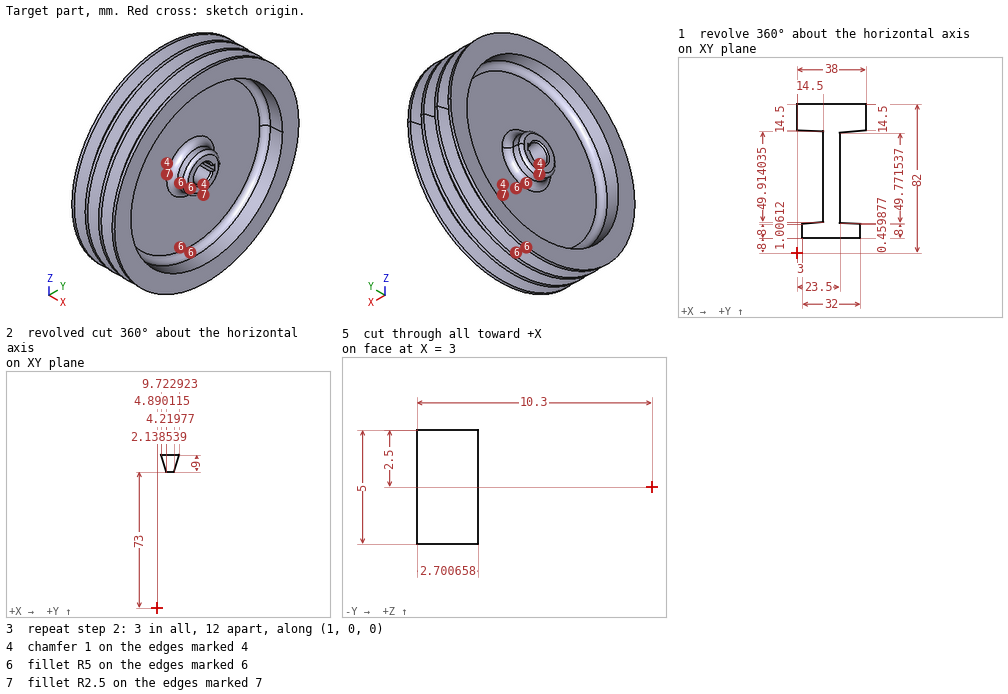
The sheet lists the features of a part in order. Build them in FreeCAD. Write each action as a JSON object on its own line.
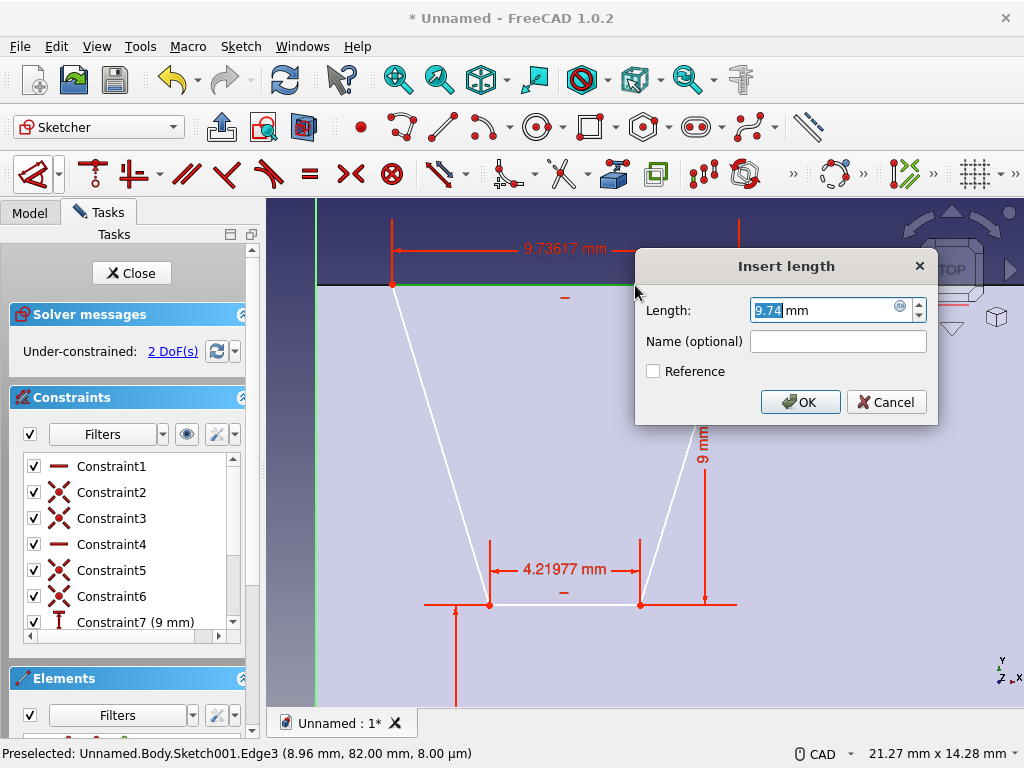
{"action": "type", "text": "9.722923"}
{"action": "key", "text": "Return"}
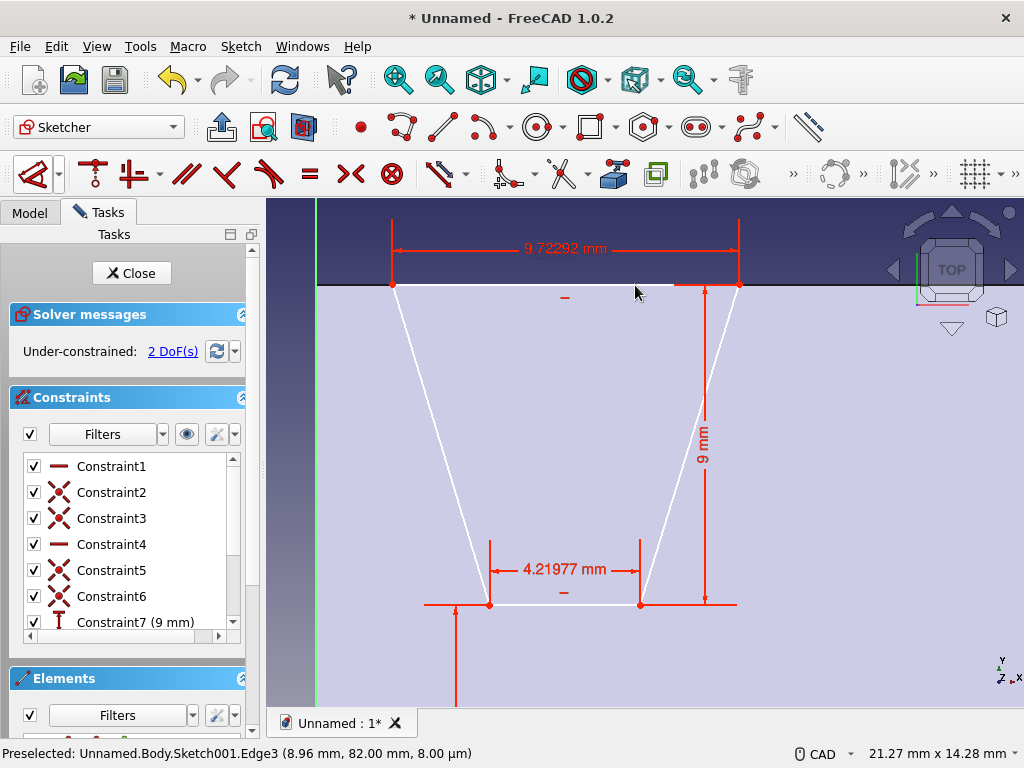
{"action": "left_click", "coordinate": [490, 605]}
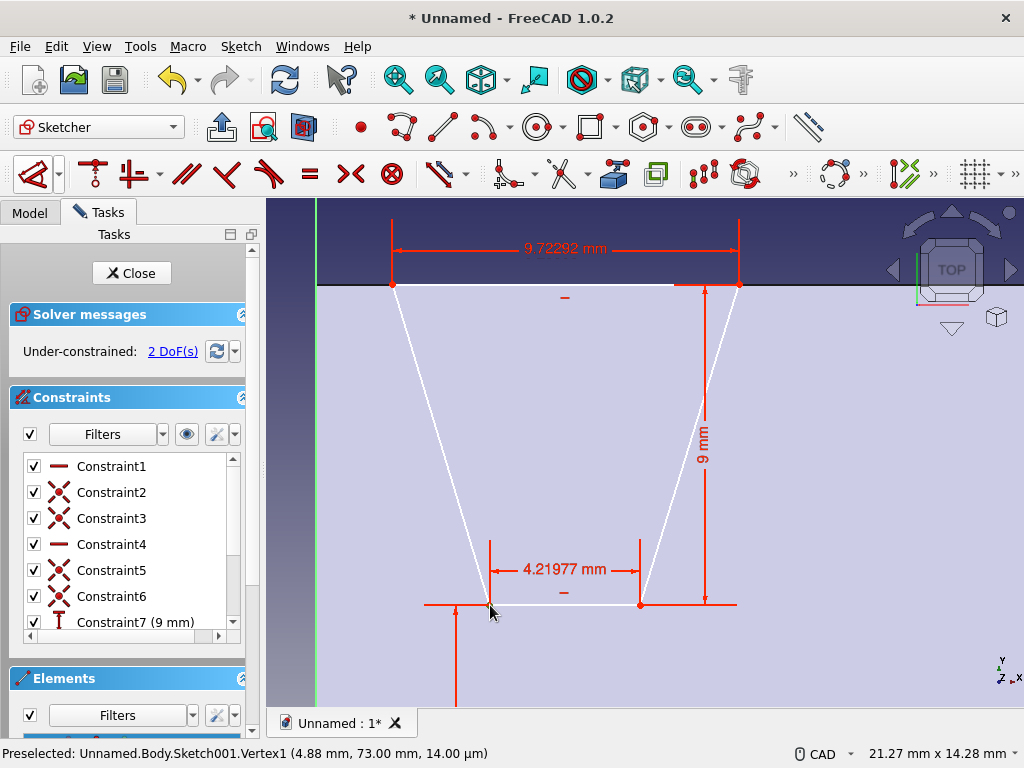
{"action": "key", "text": "l"}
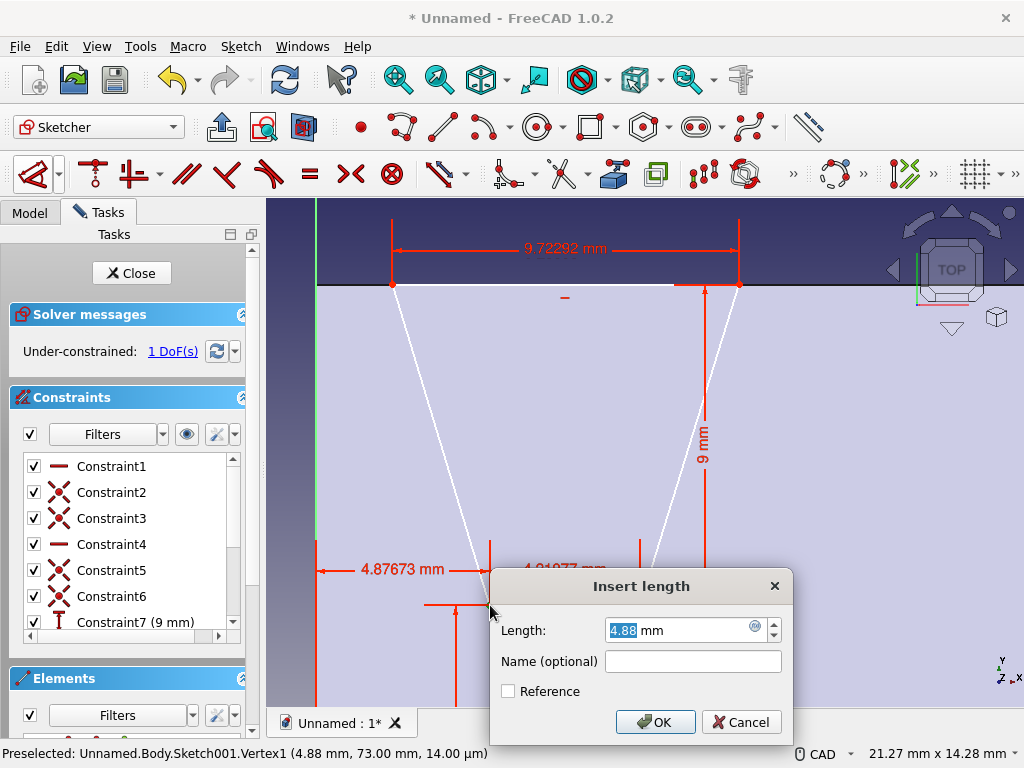
{"action": "type", "text": "4.890115"}
{"action": "key", "text": "Return"}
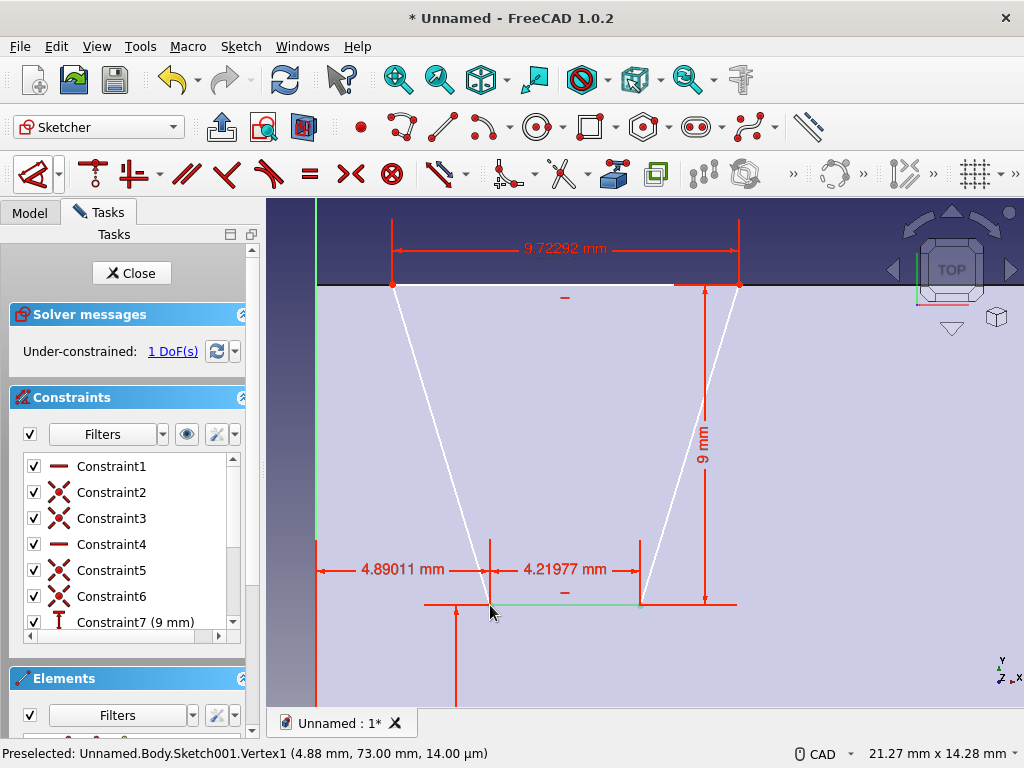
{"action": "left_click", "coordinate": [392, 285]}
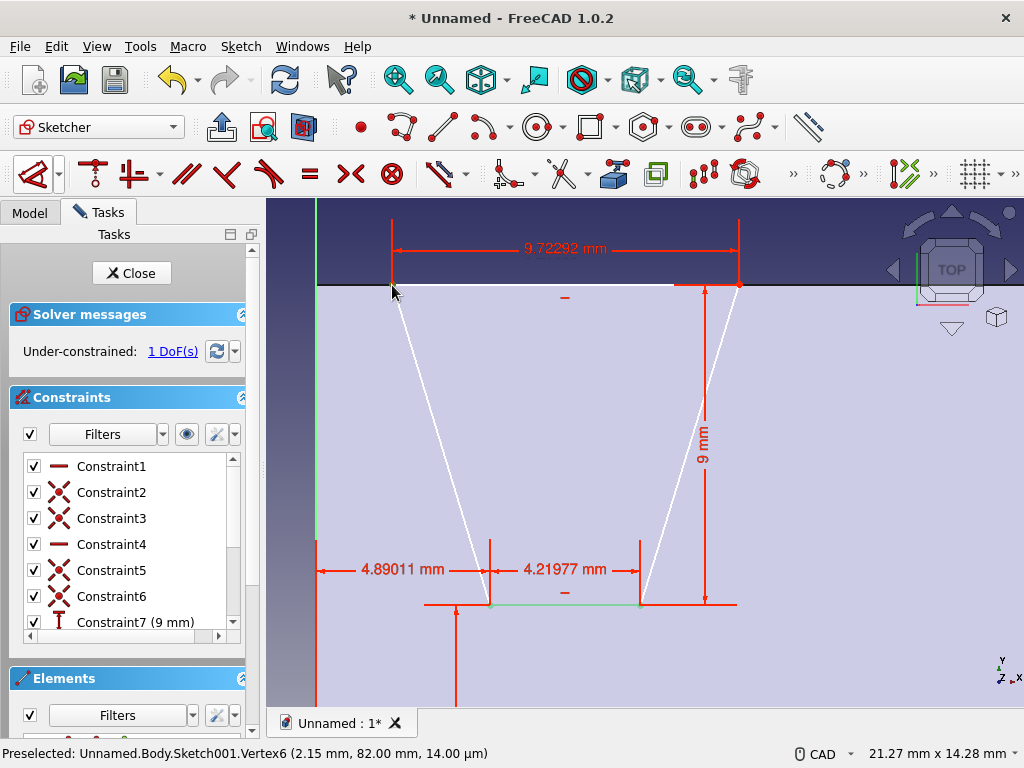
{"action": "key", "text": "l"}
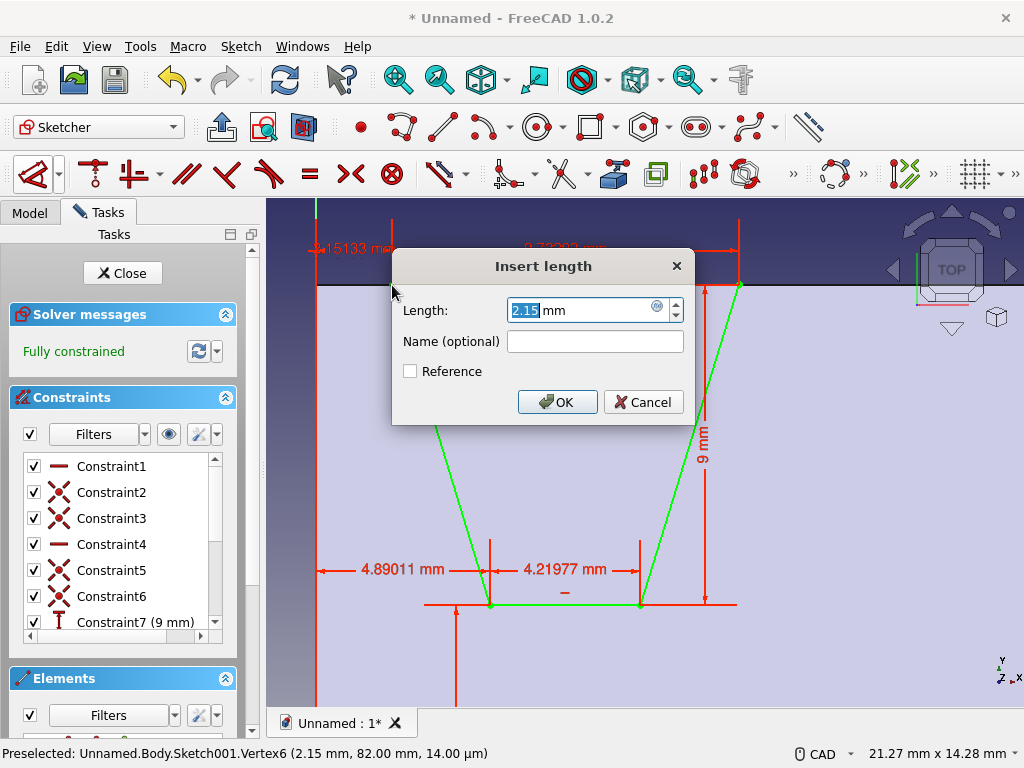
{"action": "type", "text": "2.138539"}
{"action": "key", "text": "Return"}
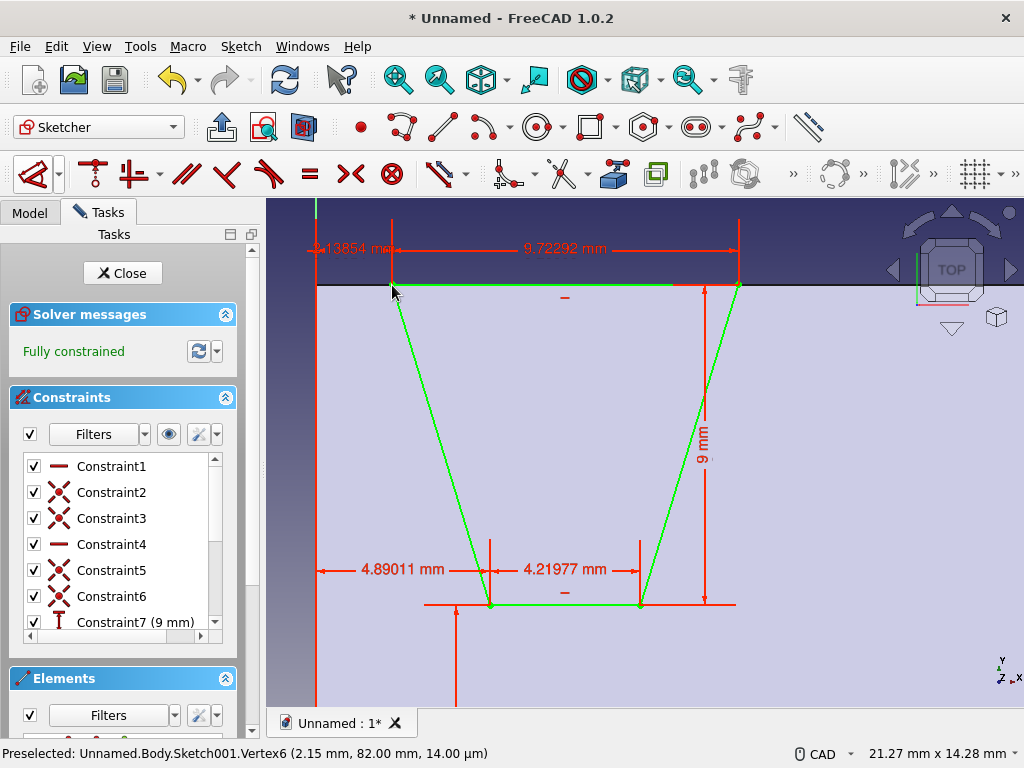
{"action": "left_click", "coordinate": [123, 273]}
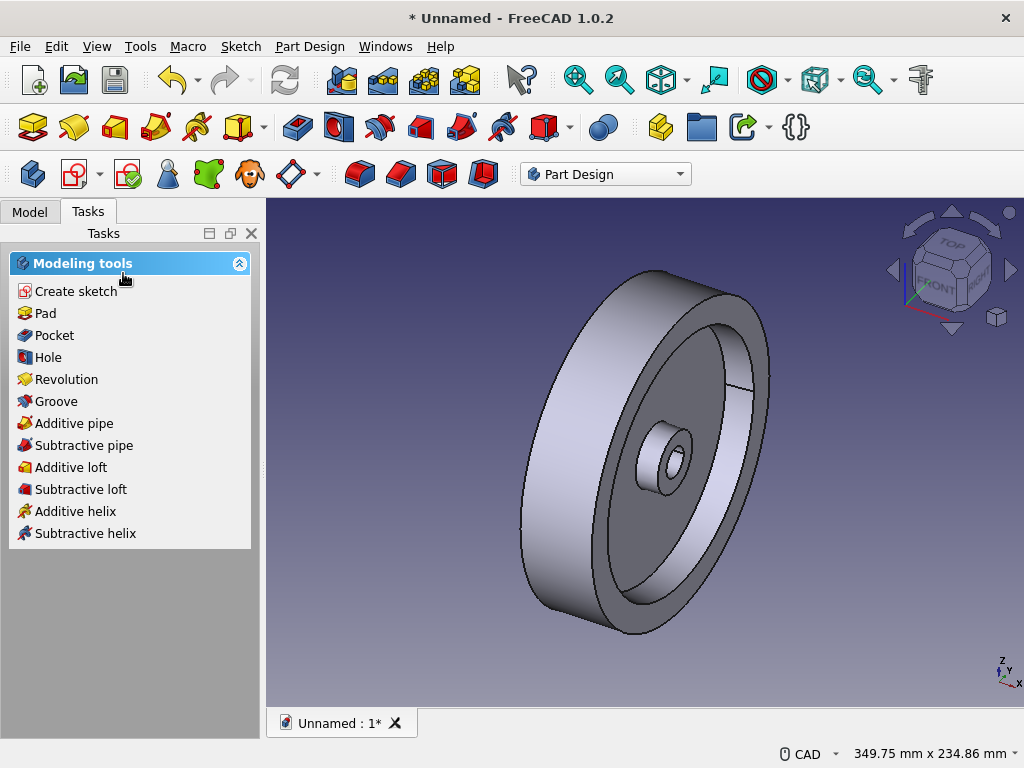
{"action": "left_click", "coordinate": [380, 128]}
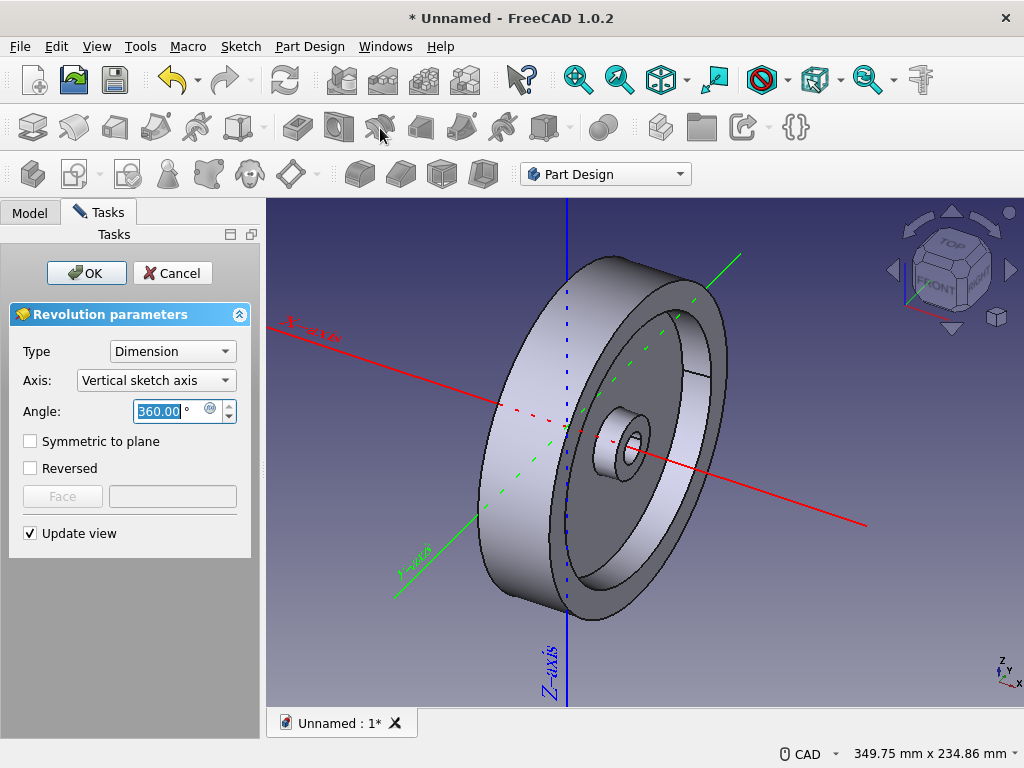
{"action": "left_click", "coordinate": [157, 380]}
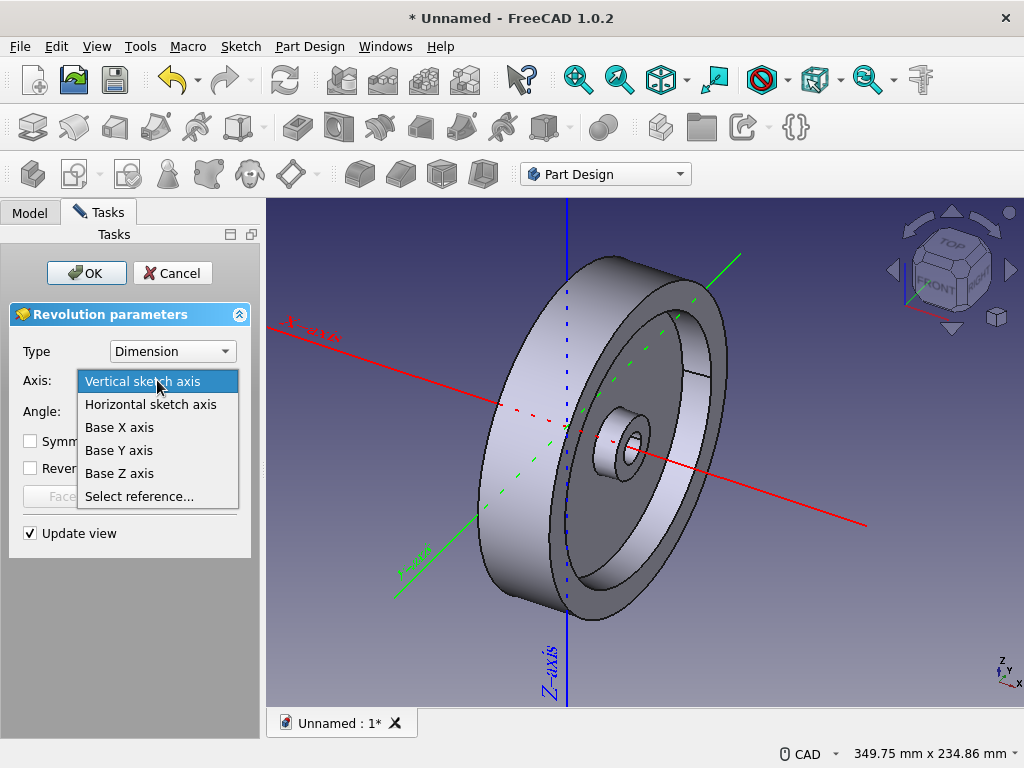
{"action": "left_click", "coordinate": [156, 404]}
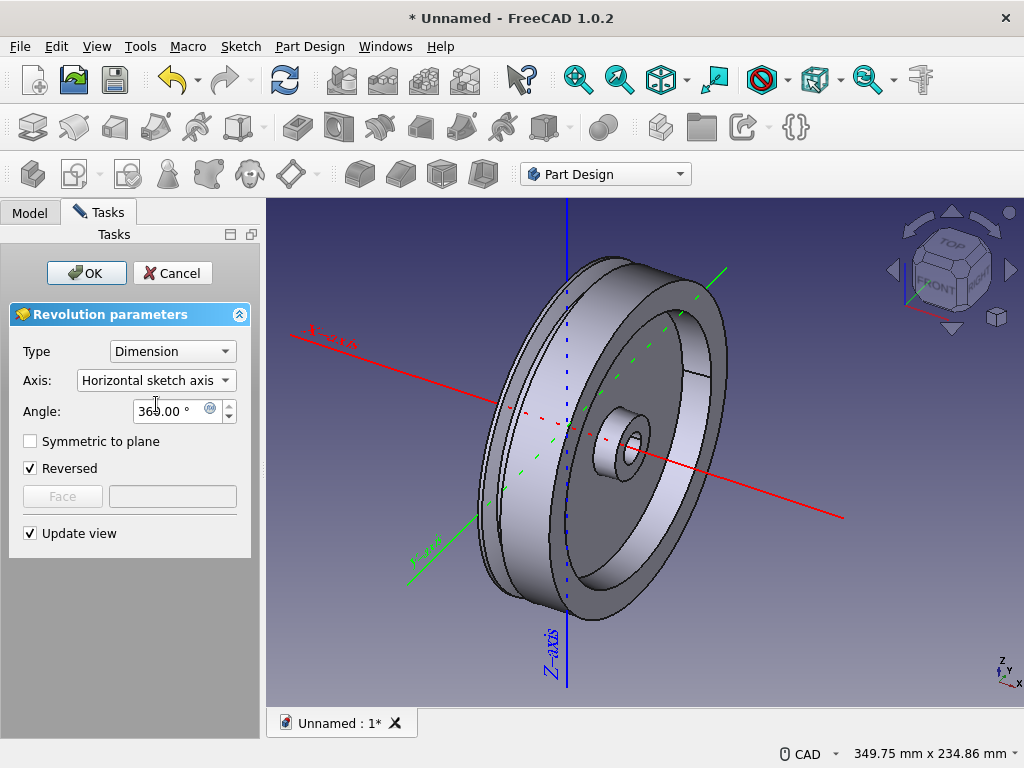
{"action": "left_click", "coordinate": [87, 273]}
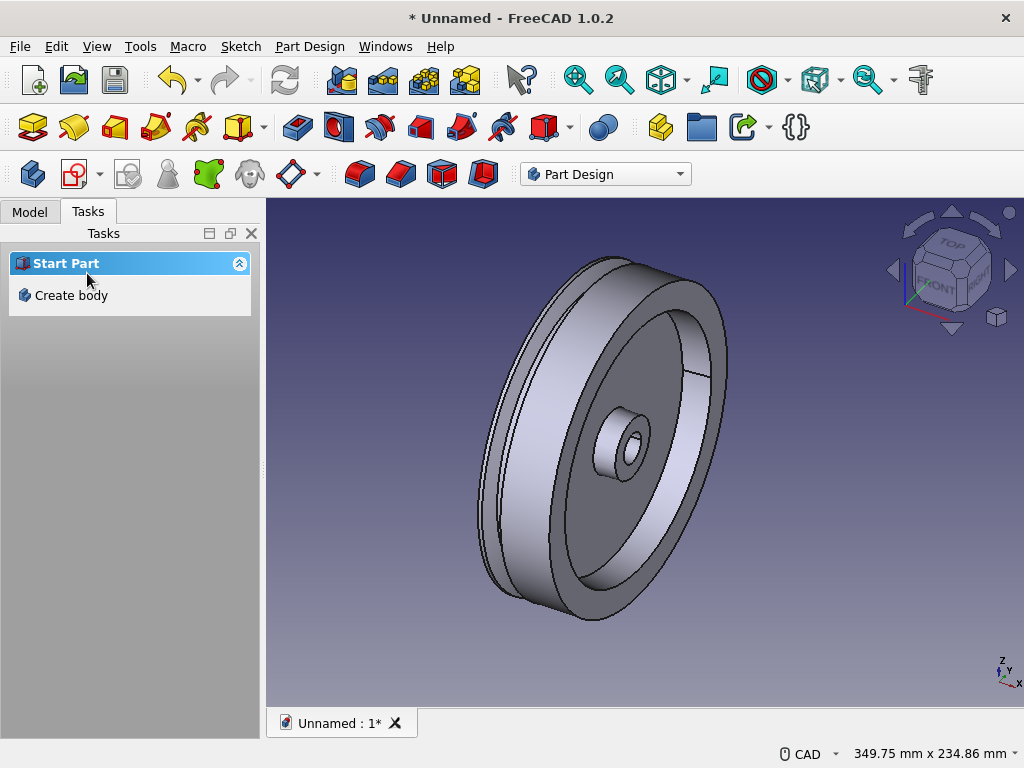
{"action": "left_click", "coordinate": [579, 80]}